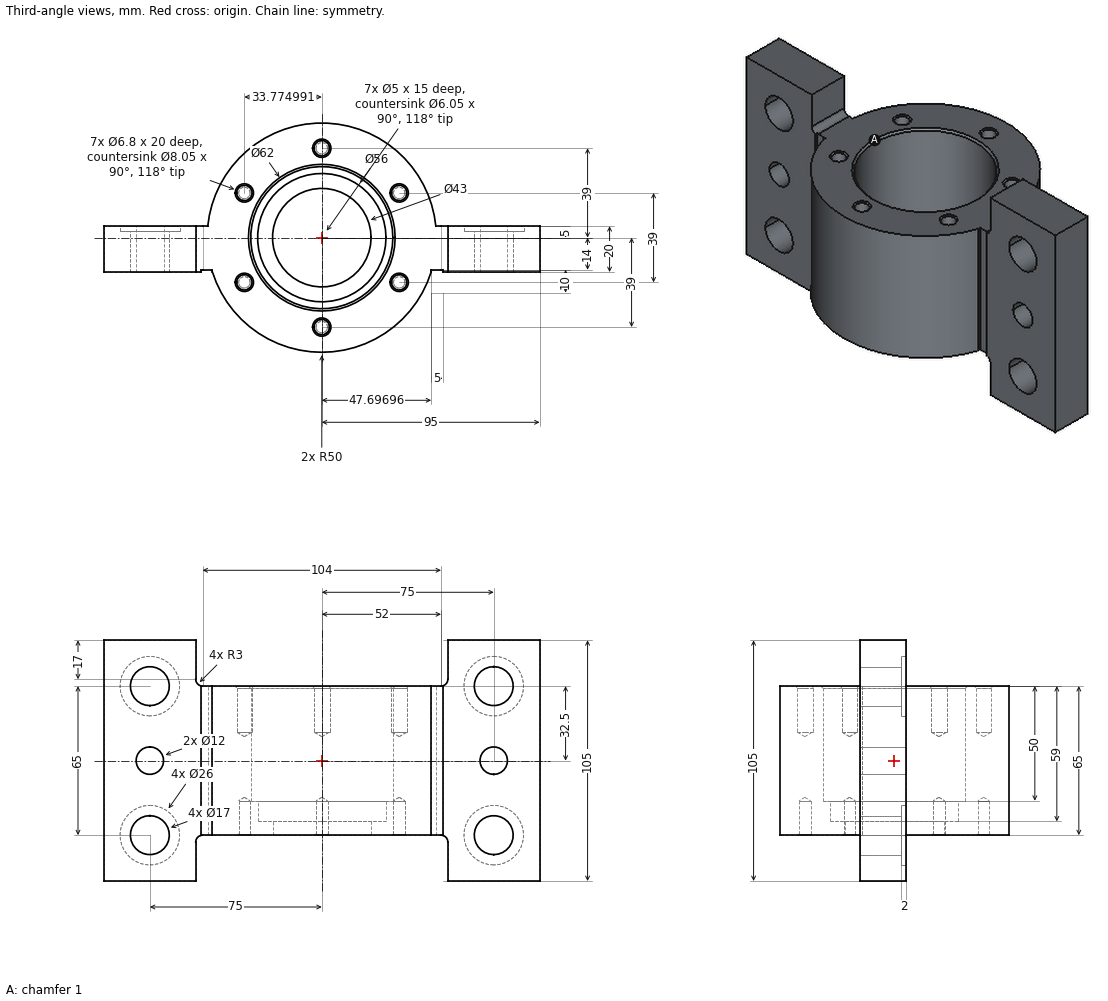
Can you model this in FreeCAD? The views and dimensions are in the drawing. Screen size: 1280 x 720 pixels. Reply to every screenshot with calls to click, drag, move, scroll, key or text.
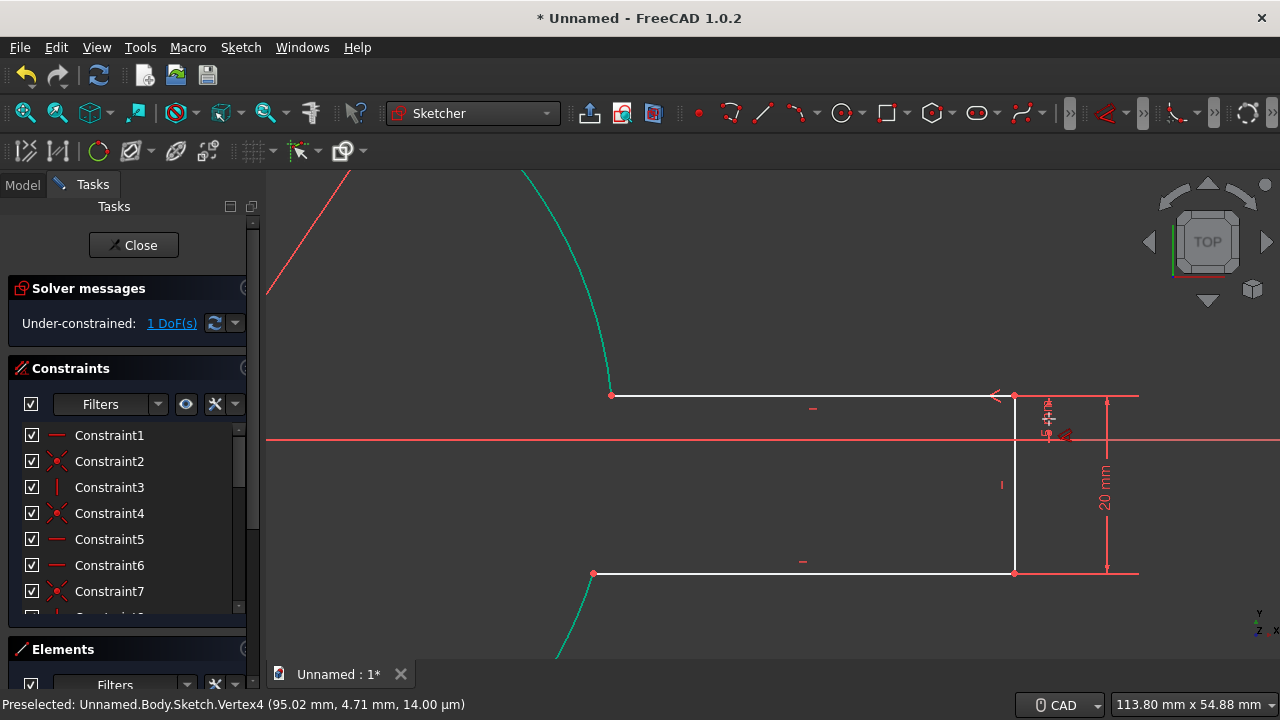
click(1015, 574)
click(654, 608)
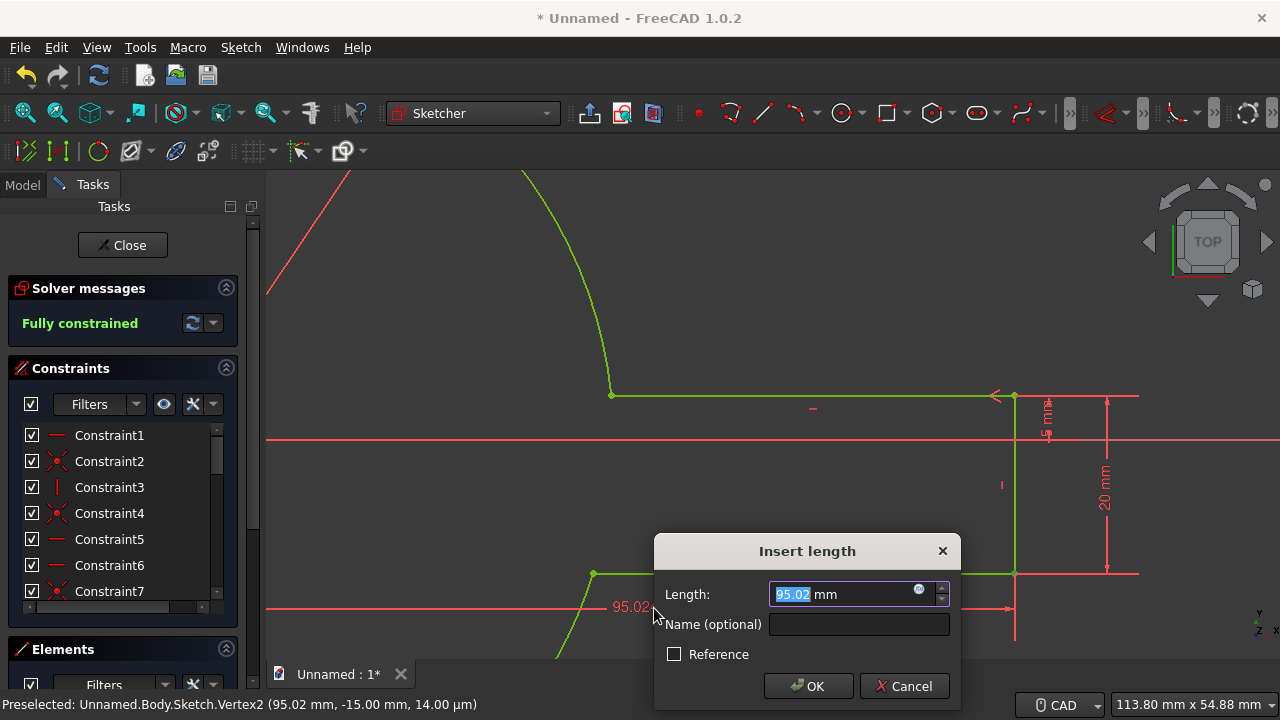
text(95)
key(Return)
key(Escape)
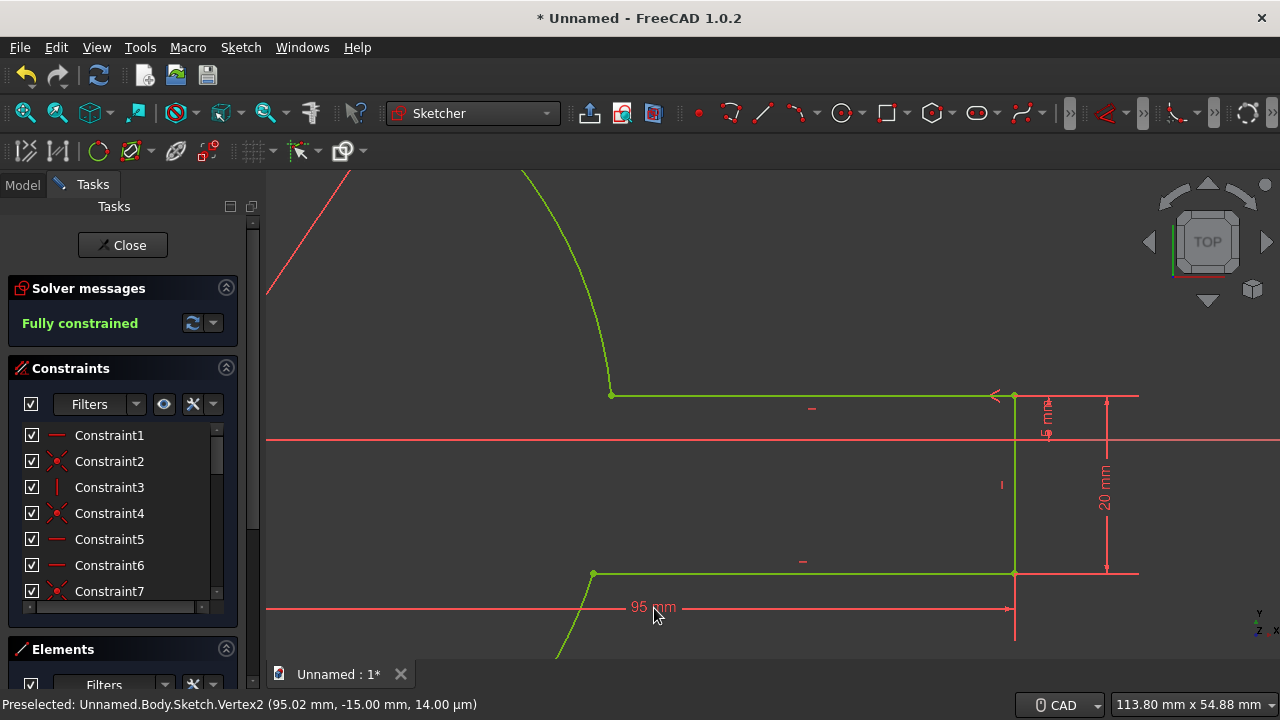
click(123, 245)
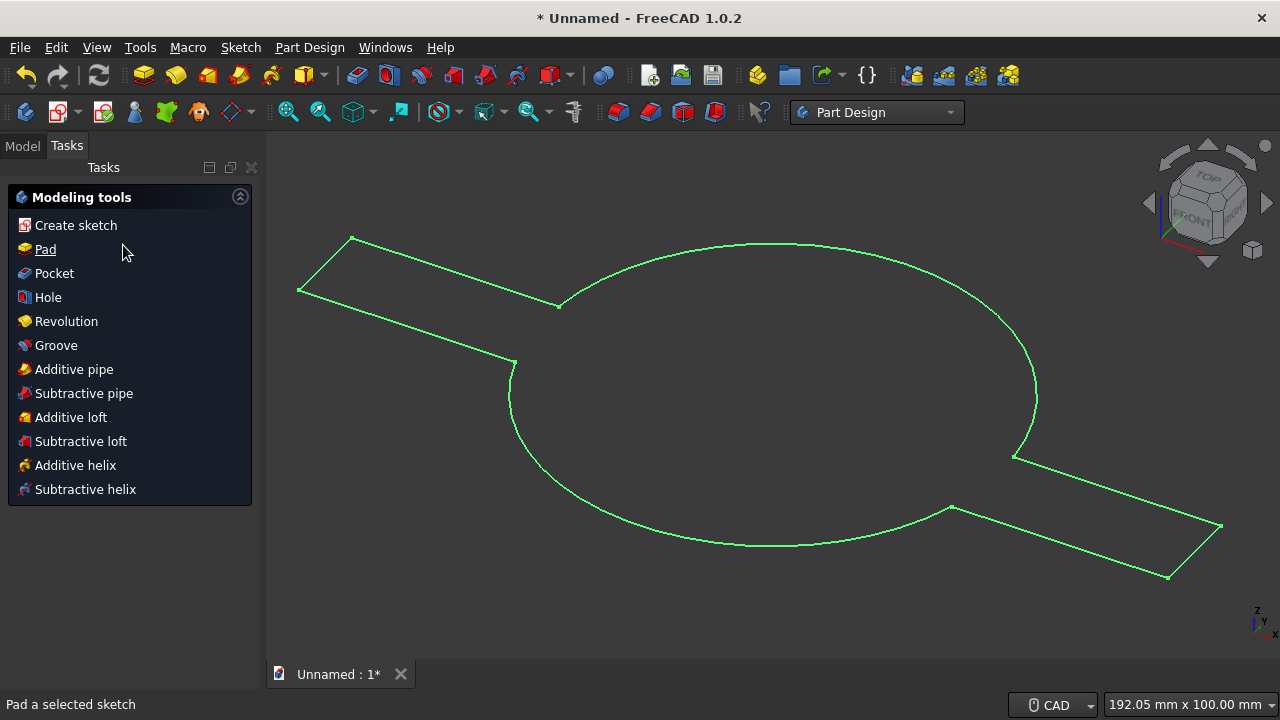
click(144, 76)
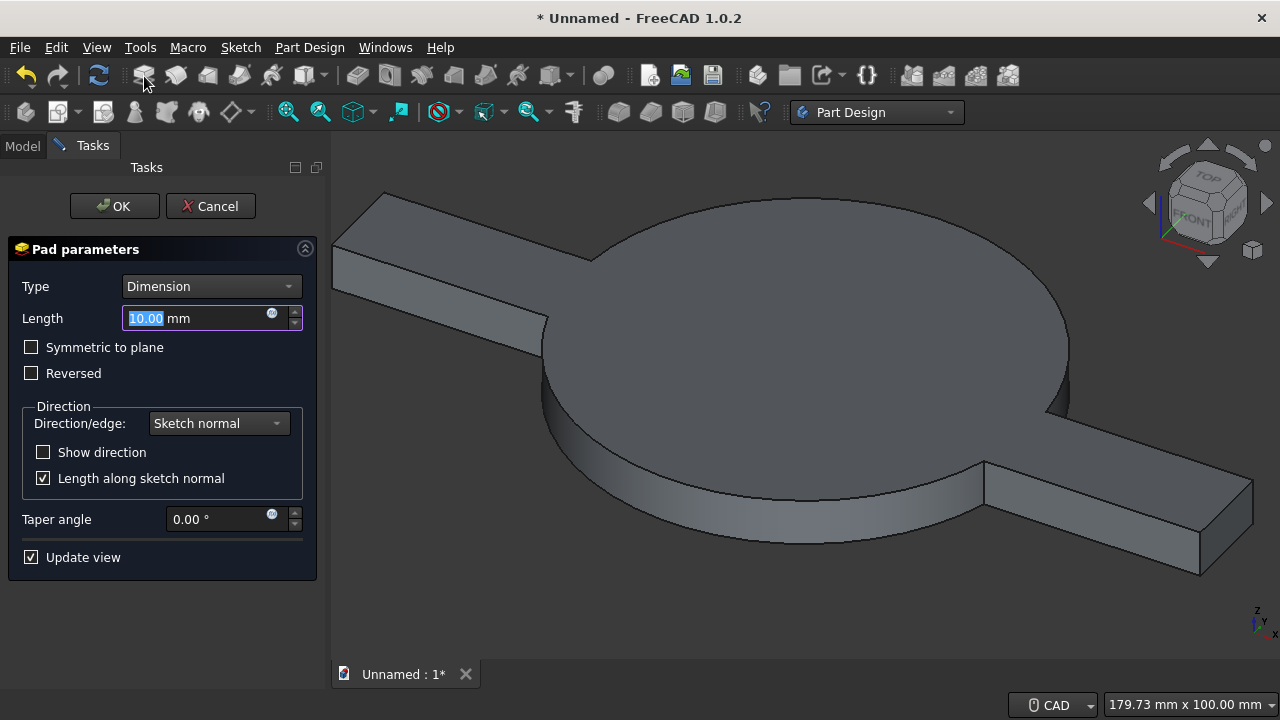
text(105)
key(Tab)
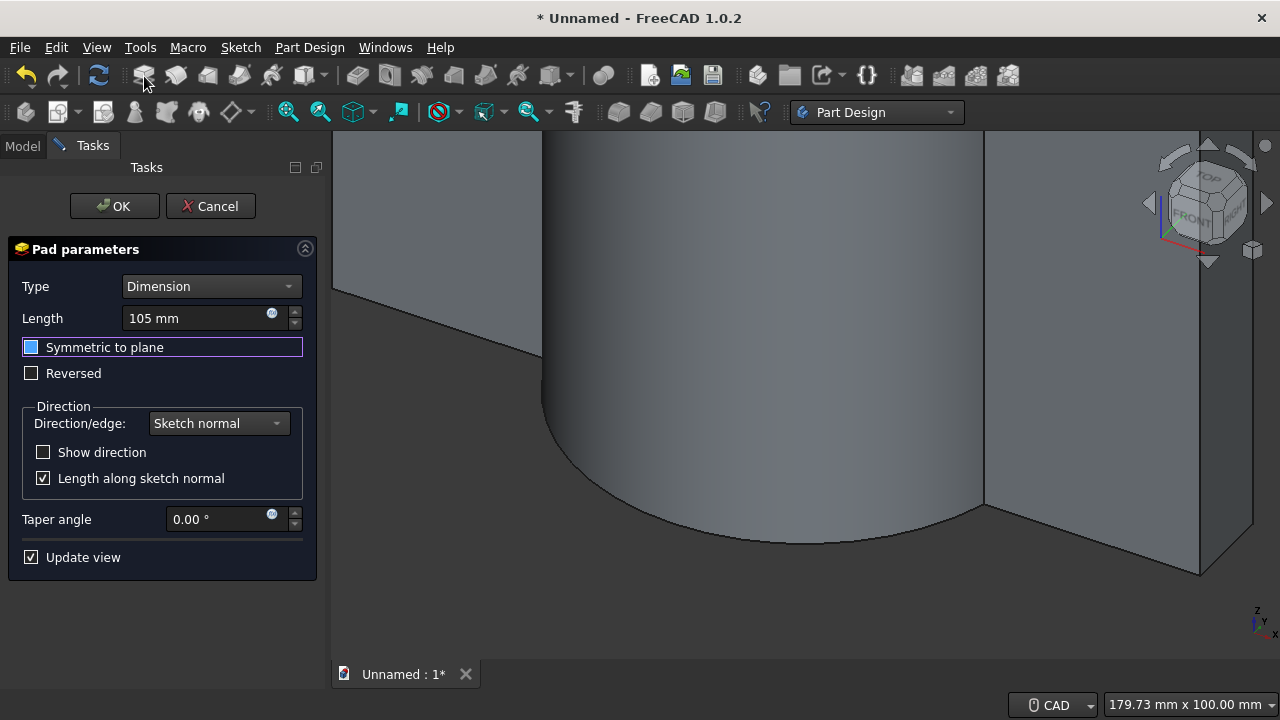
click(30, 347)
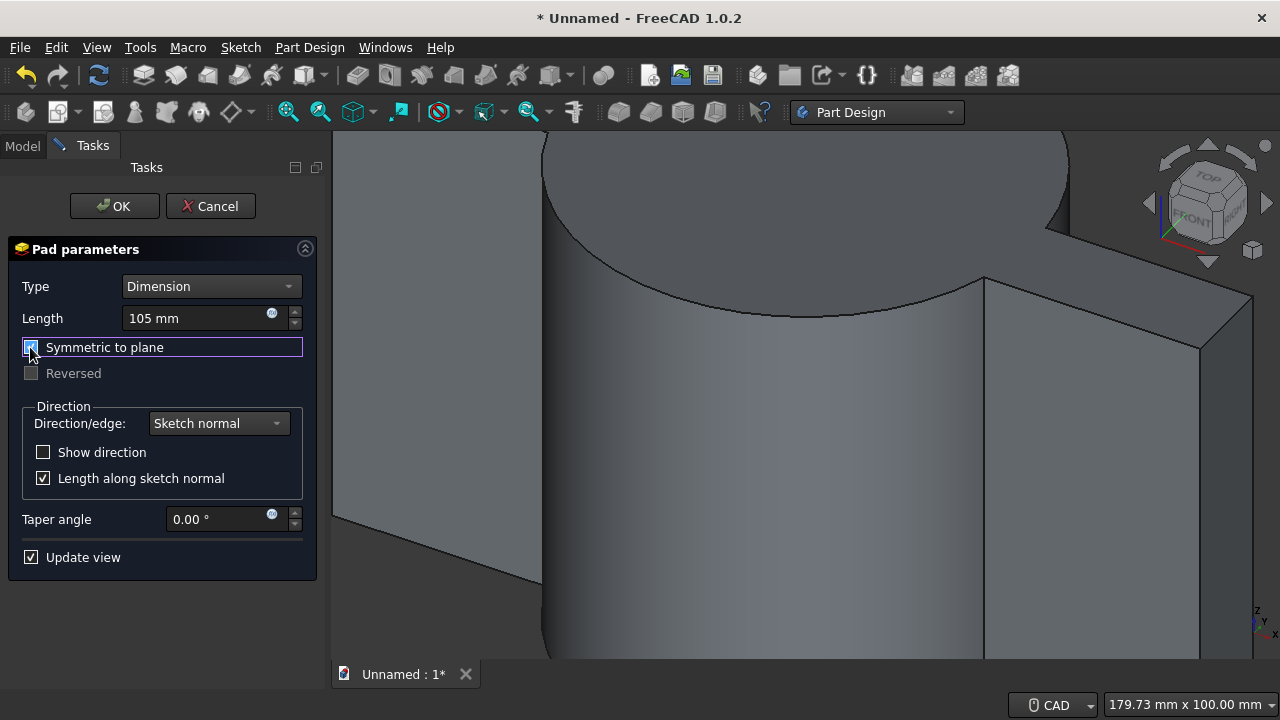
click(115, 206)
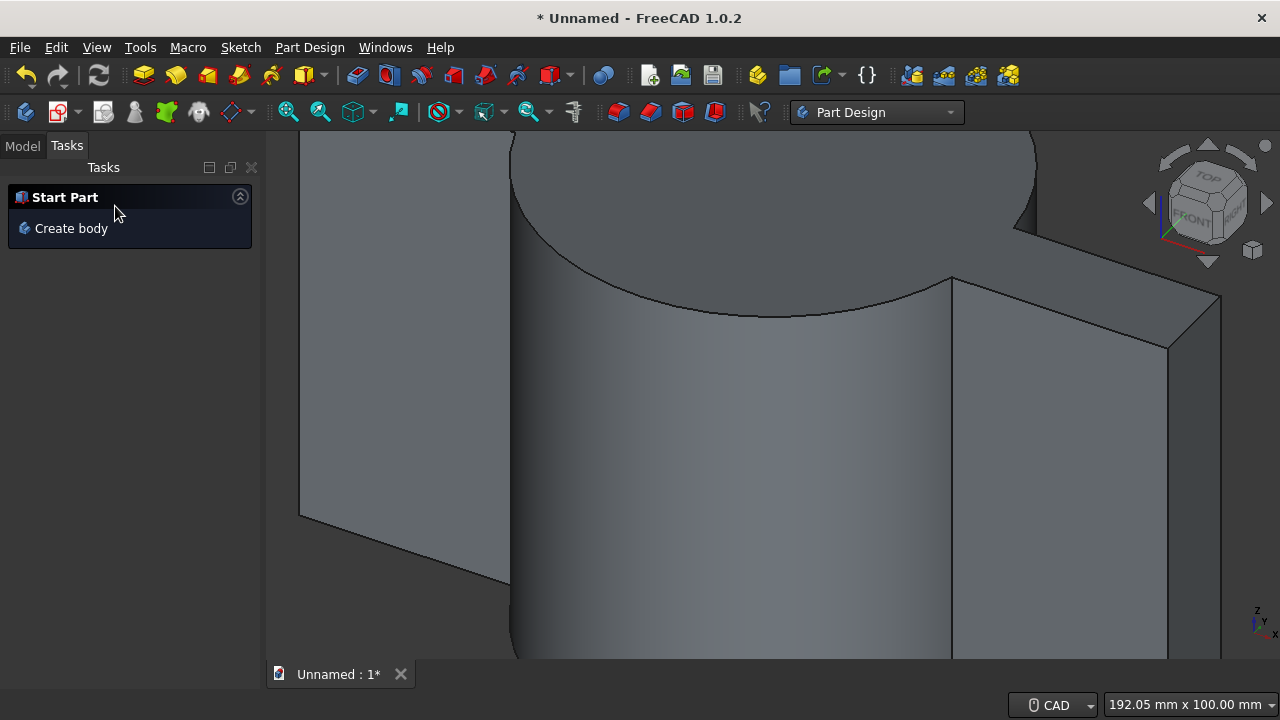
click(290, 112)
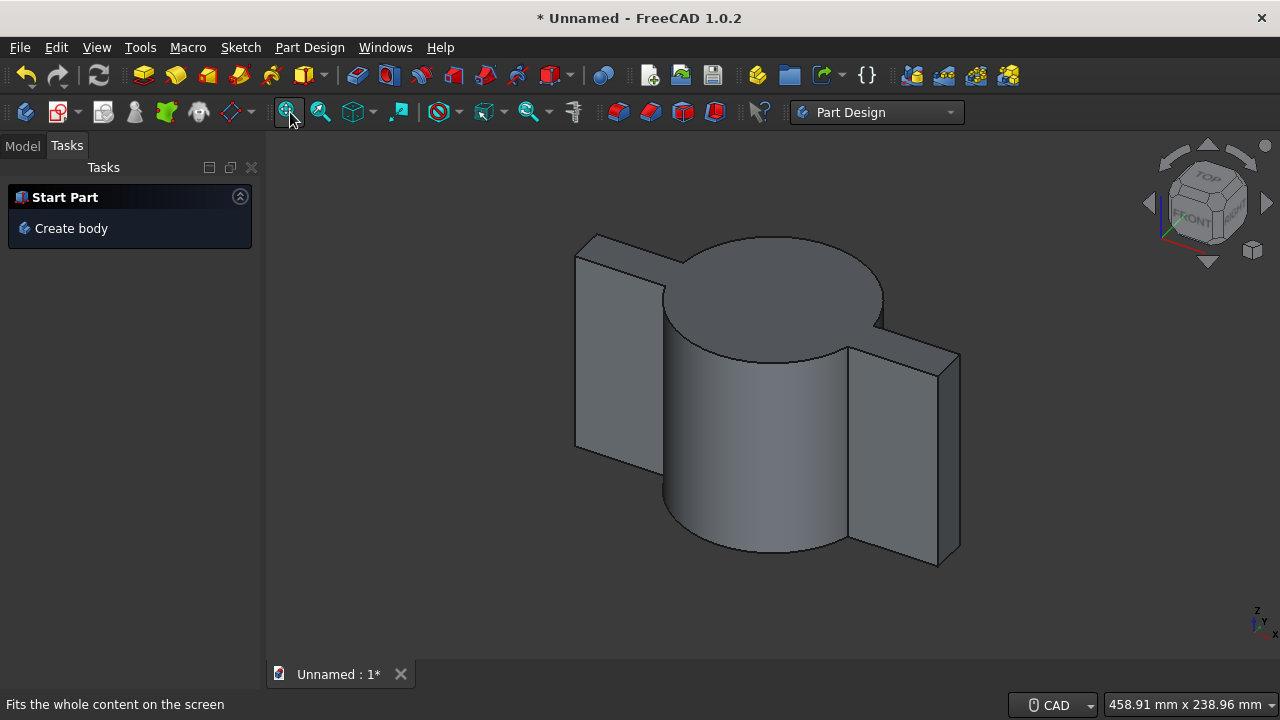
click(773, 299)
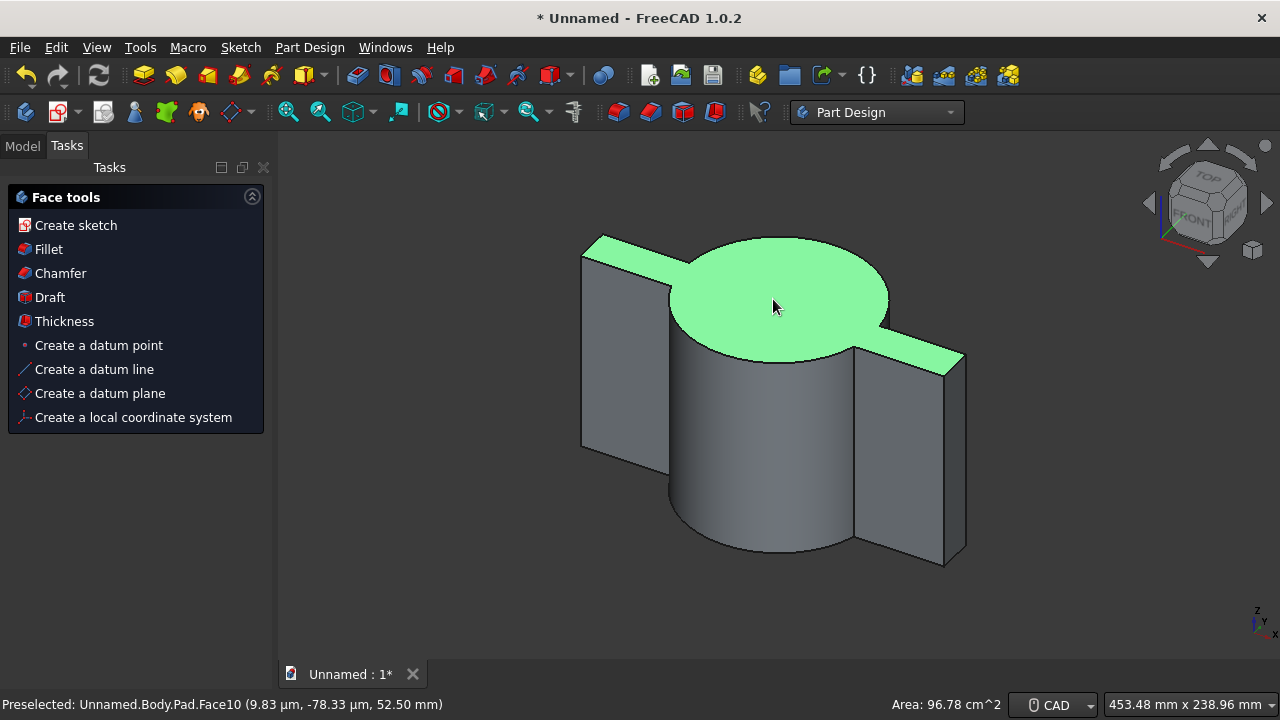
click(58, 112)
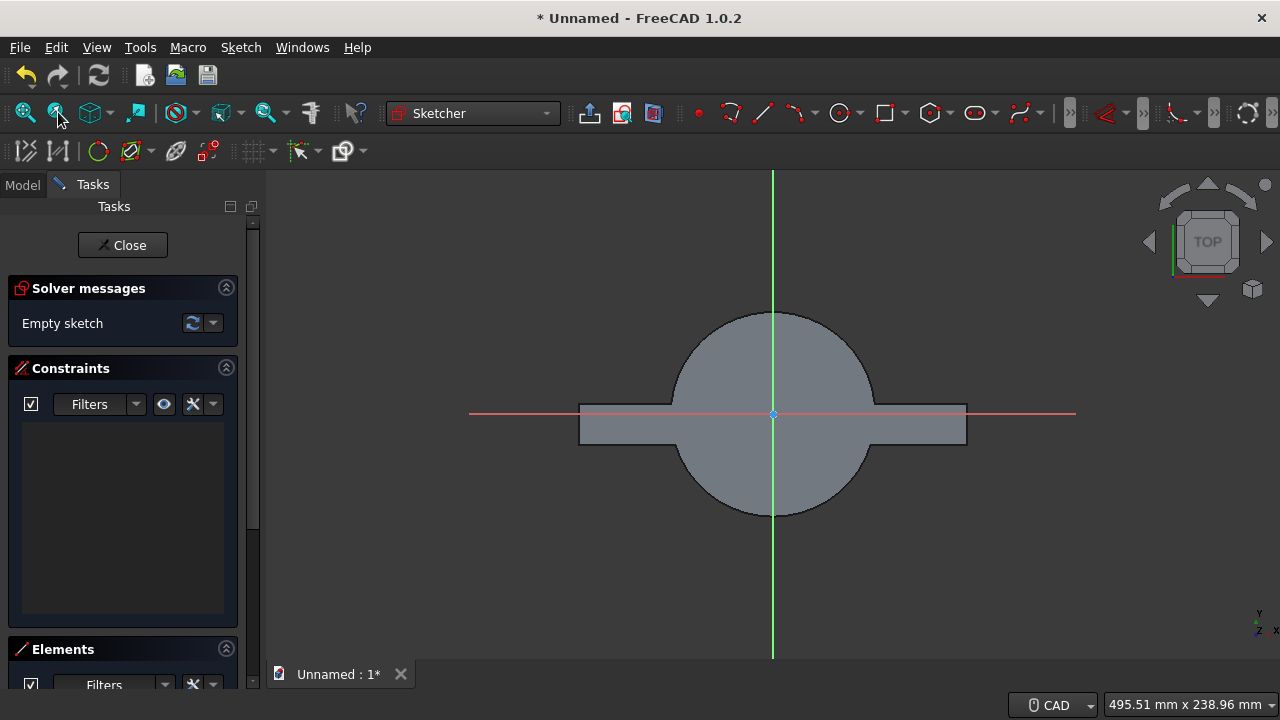
scroll(813, 453, up, 5)